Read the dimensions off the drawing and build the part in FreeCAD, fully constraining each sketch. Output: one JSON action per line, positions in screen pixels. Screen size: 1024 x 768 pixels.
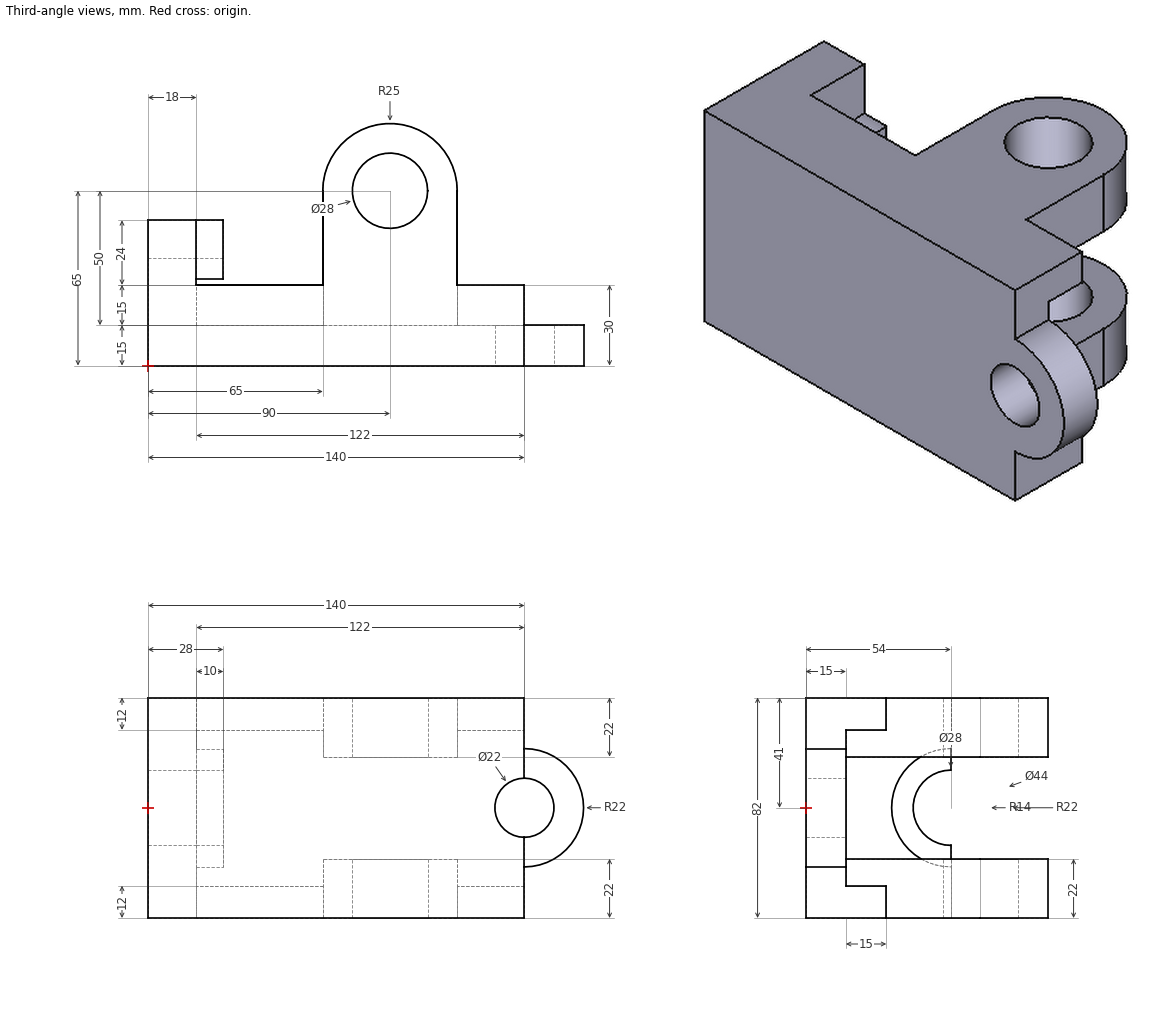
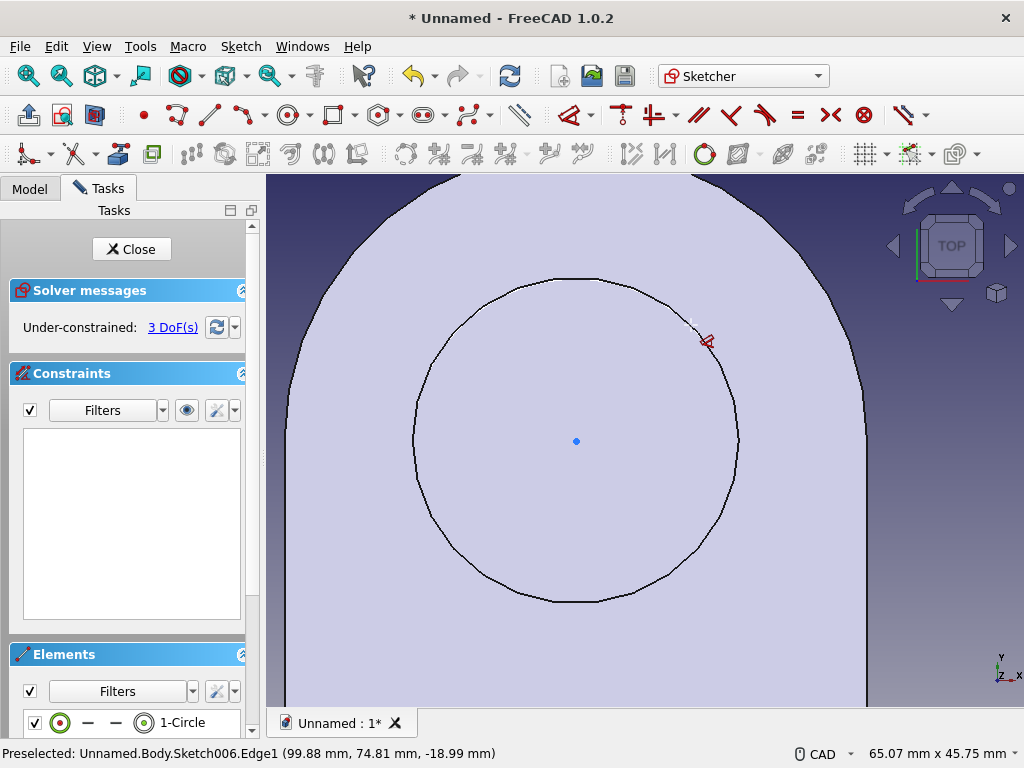
{"action": "left_click", "coordinate": [691, 326]}
{"action": "left_click", "coordinate": [714, 303]}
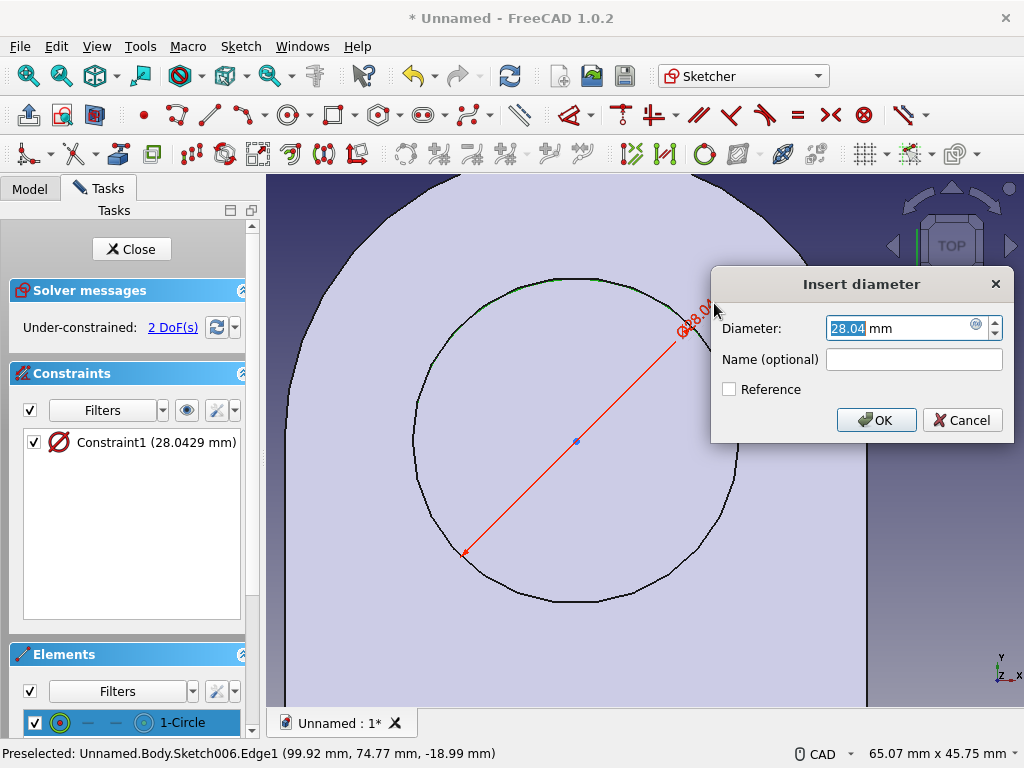
{"action": "type", "text": "28"}
{"action": "key", "text": "Return"}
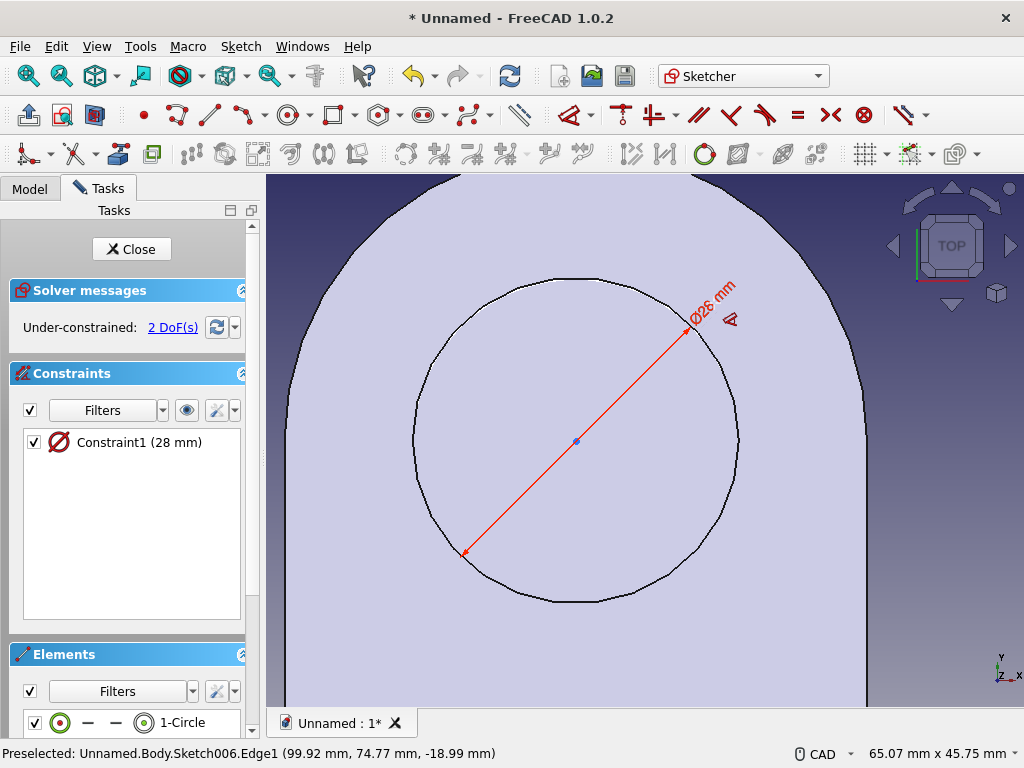
{"action": "left_click", "coordinate": [576, 442]}
{"action": "left_click", "coordinate": [435, 408]}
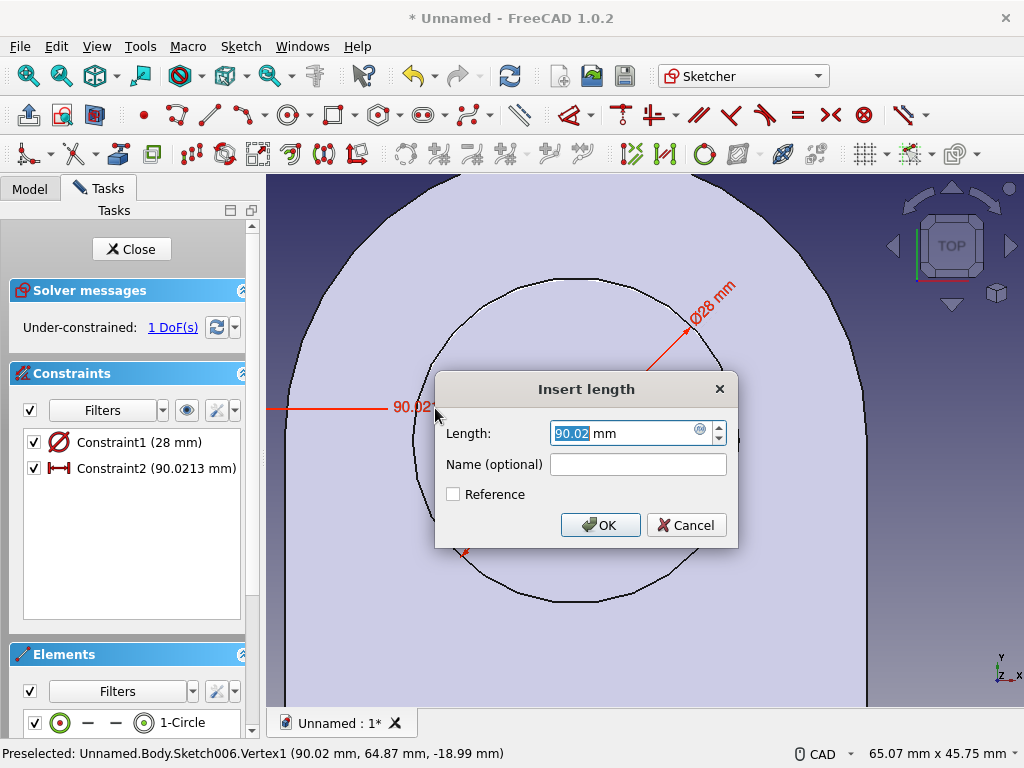
{"action": "type", "text": "90"}
{"action": "key", "text": "Return"}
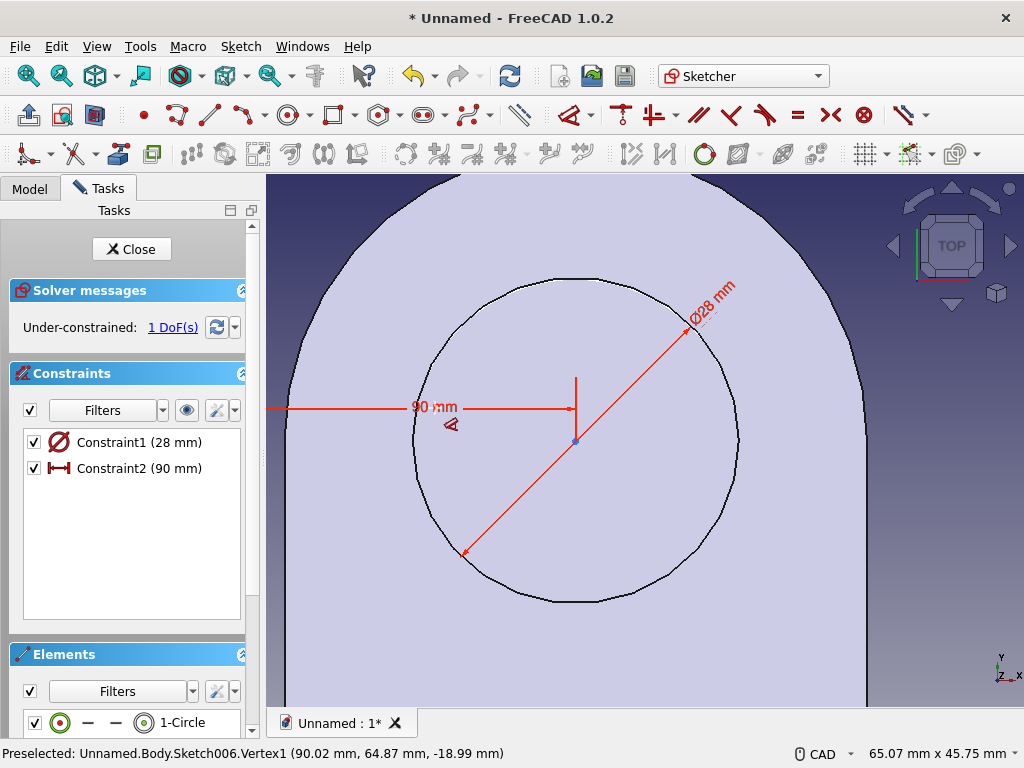
{"action": "left_click", "coordinate": [576, 442]}
{"action": "left_click", "coordinate": [610, 561]}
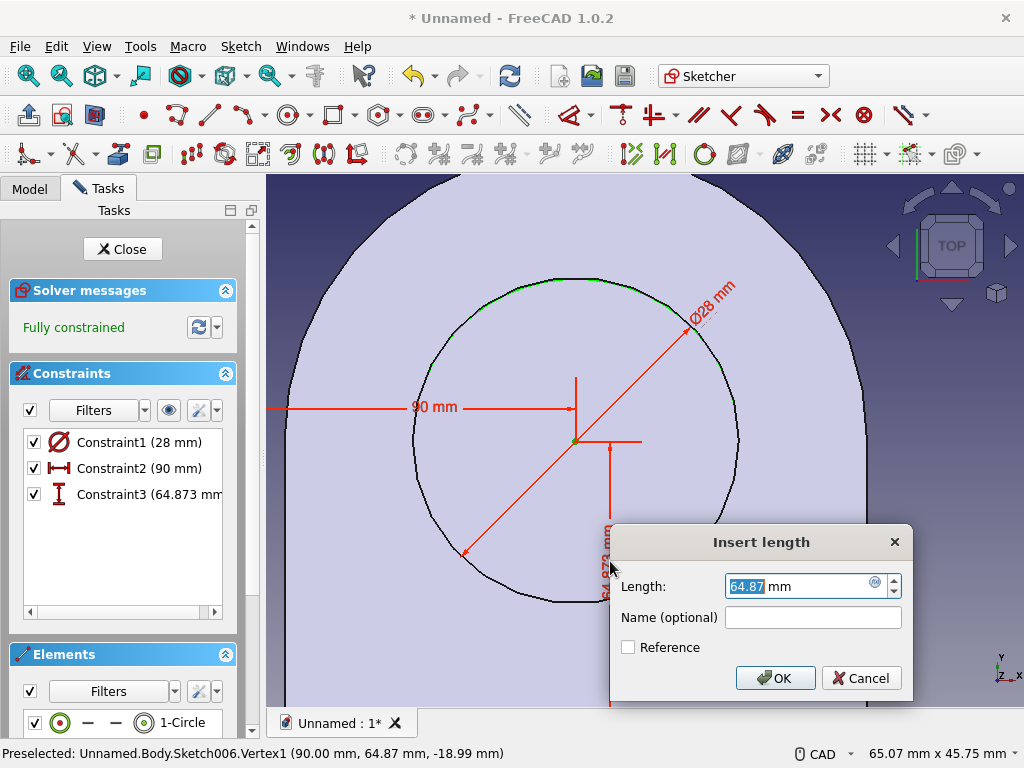
{"action": "type", "text": "65"}
{"action": "key", "text": "Return"}
{"action": "key", "text": "Escape"}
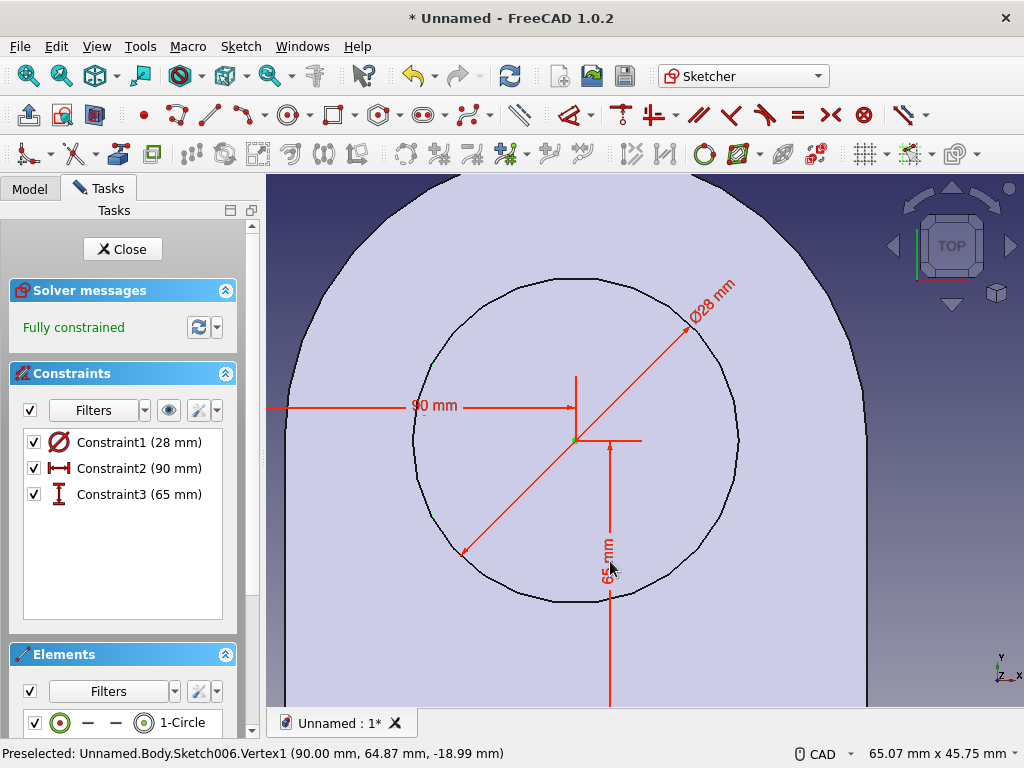
{"action": "left_click", "coordinate": [123, 249]}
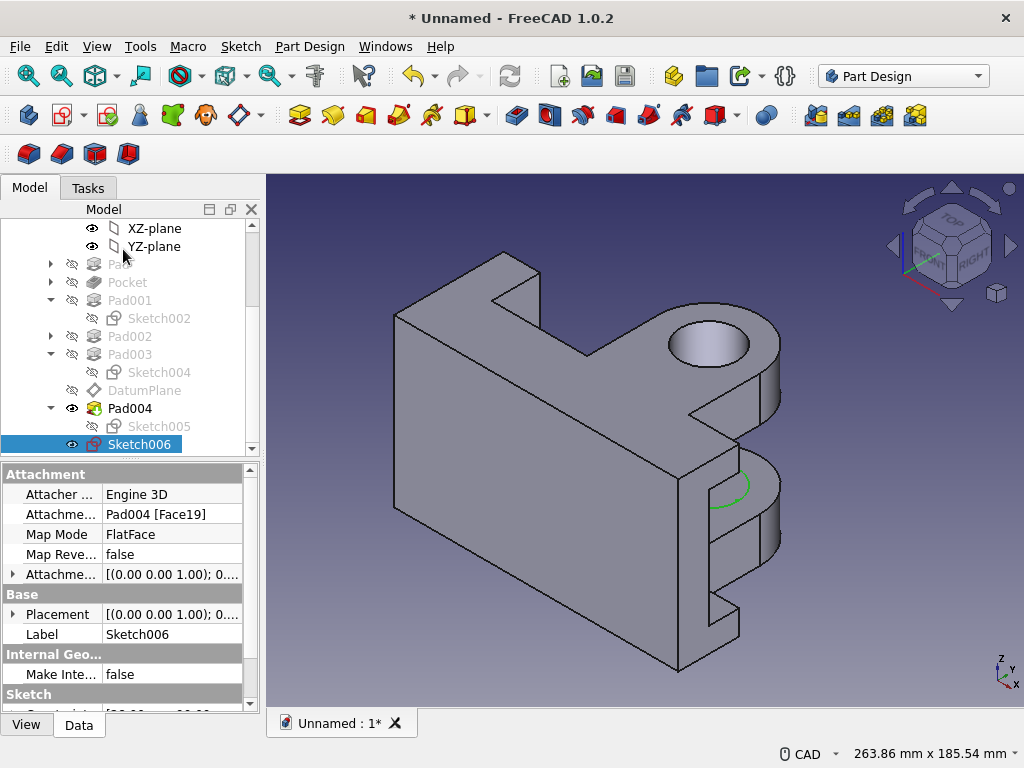
{"action": "left_click", "coordinate": [517, 116]}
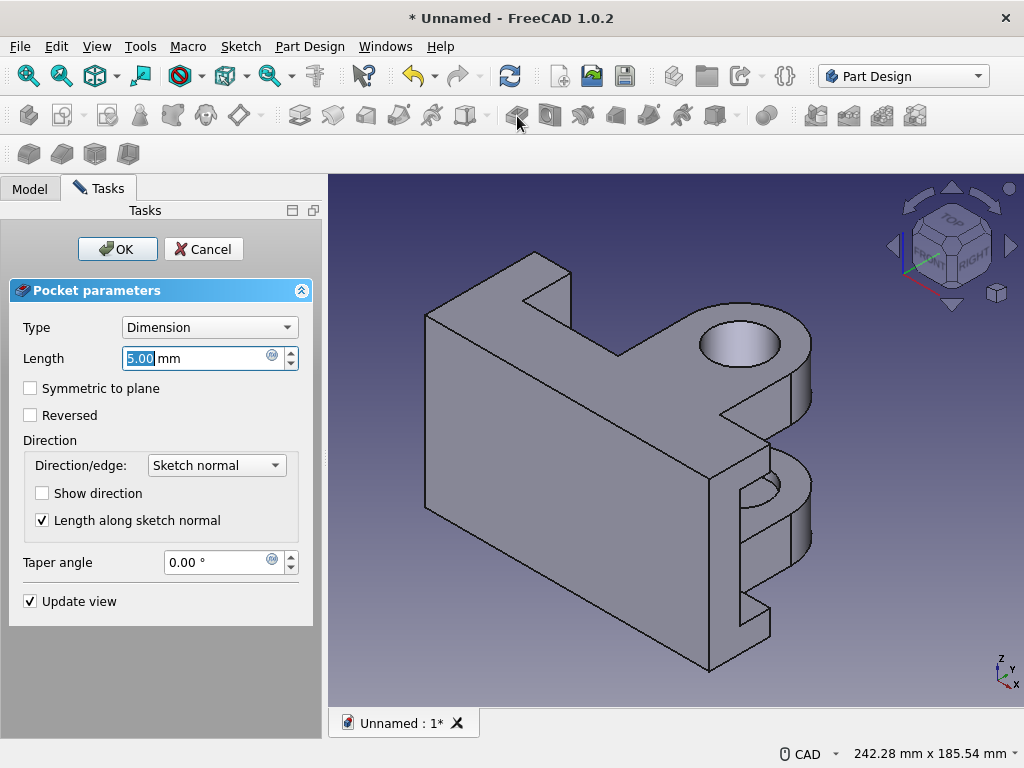
{"action": "type", "text": "22"}
{"action": "key", "text": "Tab"}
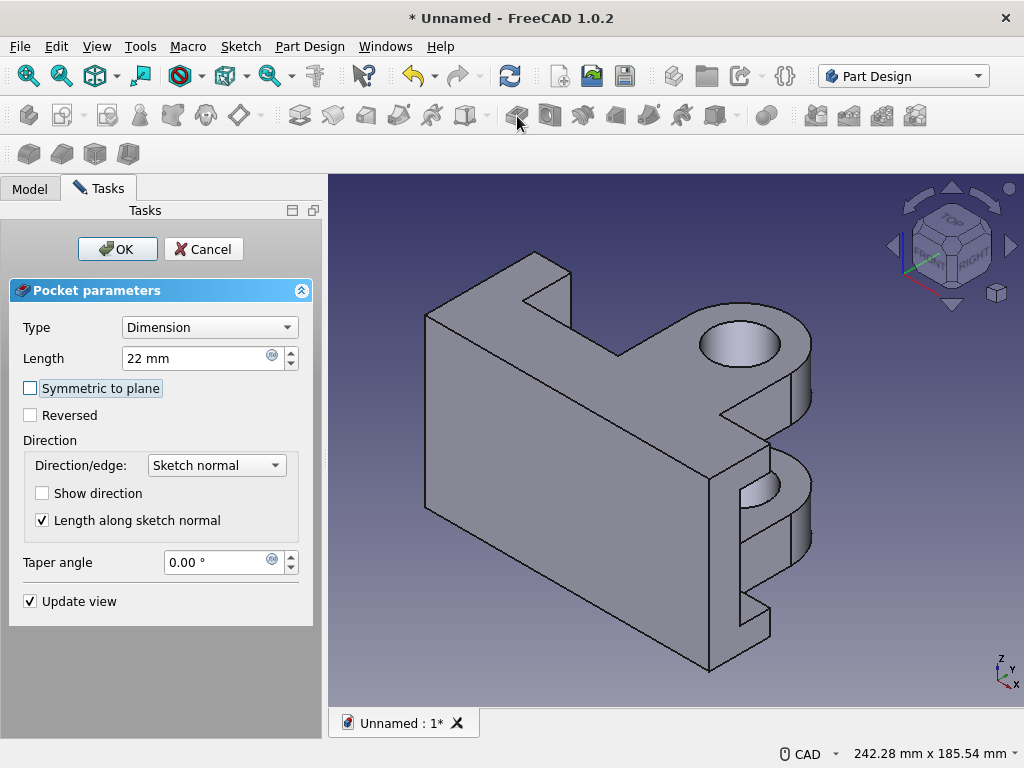
{"action": "left_click", "coordinate": [118, 249]}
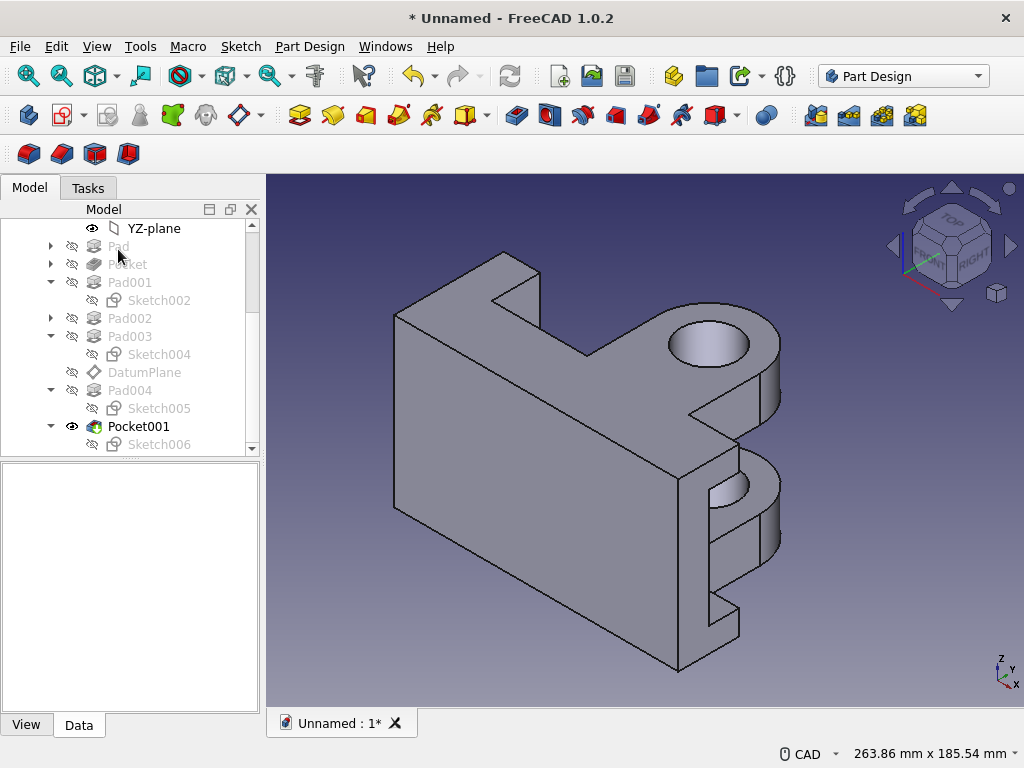
{"action": "key", "text": "3"}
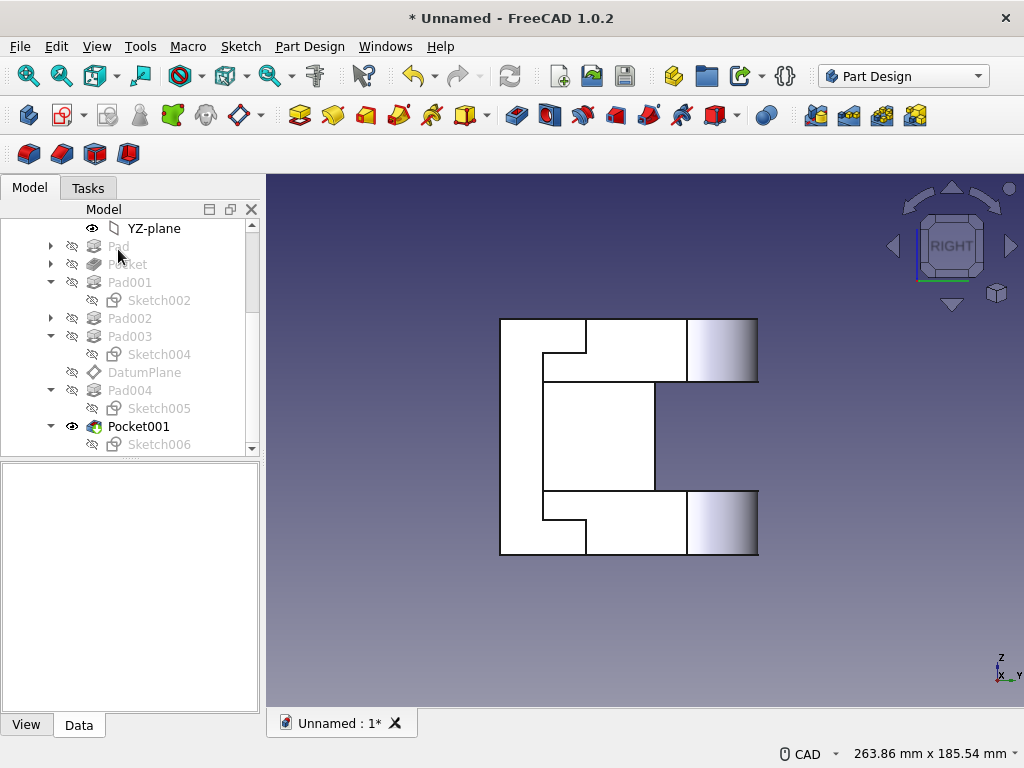
{"action": "key", "text": "v f"}